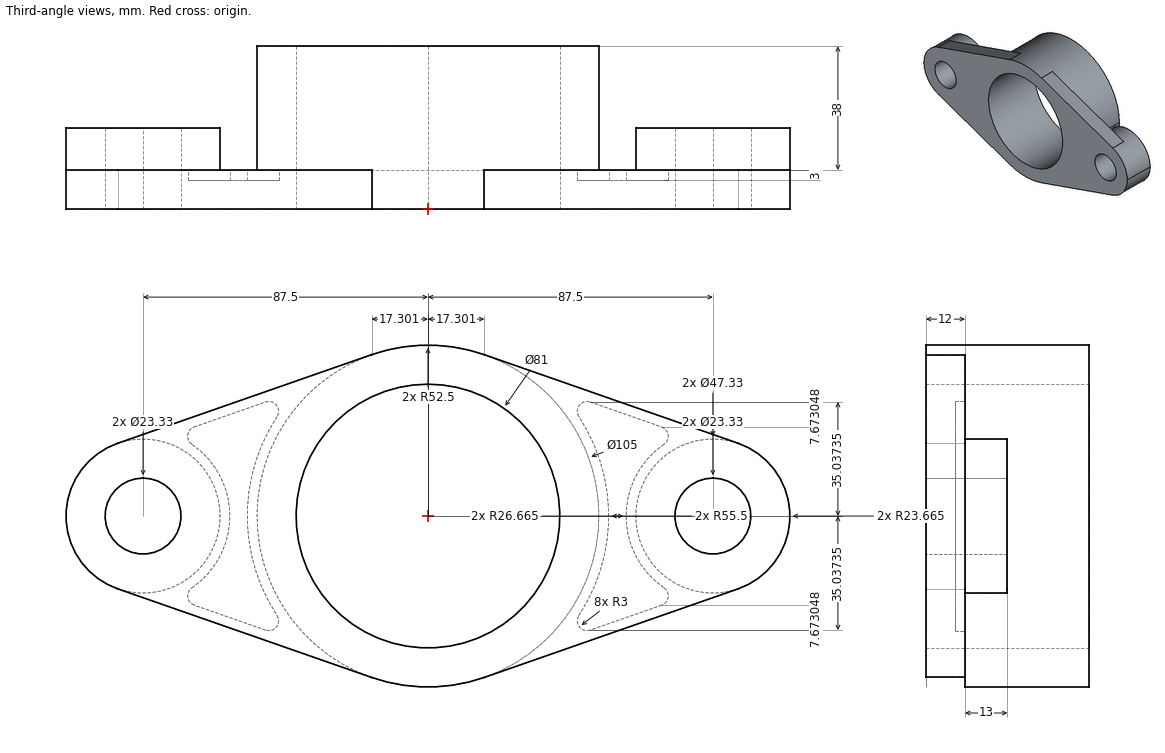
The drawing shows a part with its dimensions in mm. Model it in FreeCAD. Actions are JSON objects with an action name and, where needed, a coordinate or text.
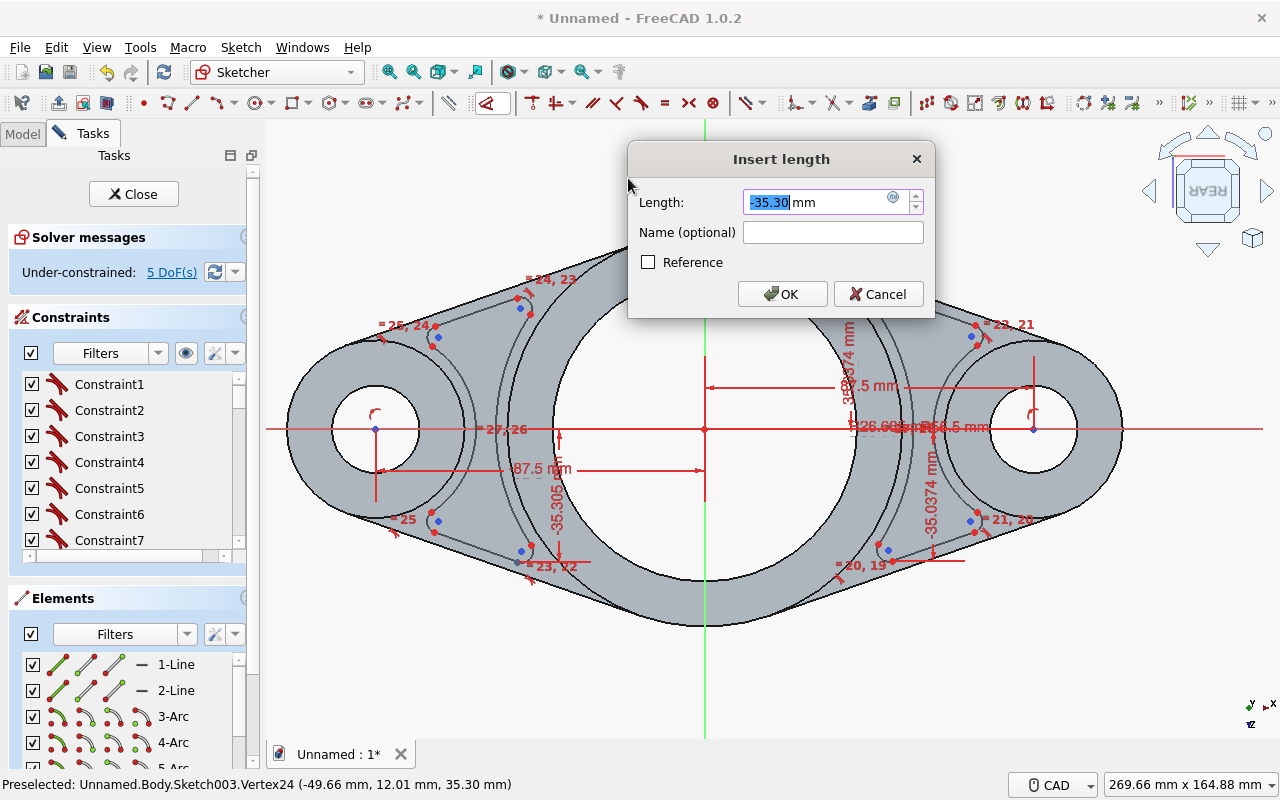
{"action": "type", "text": "-35.03735"}
{"action": "key", "text": "Return"}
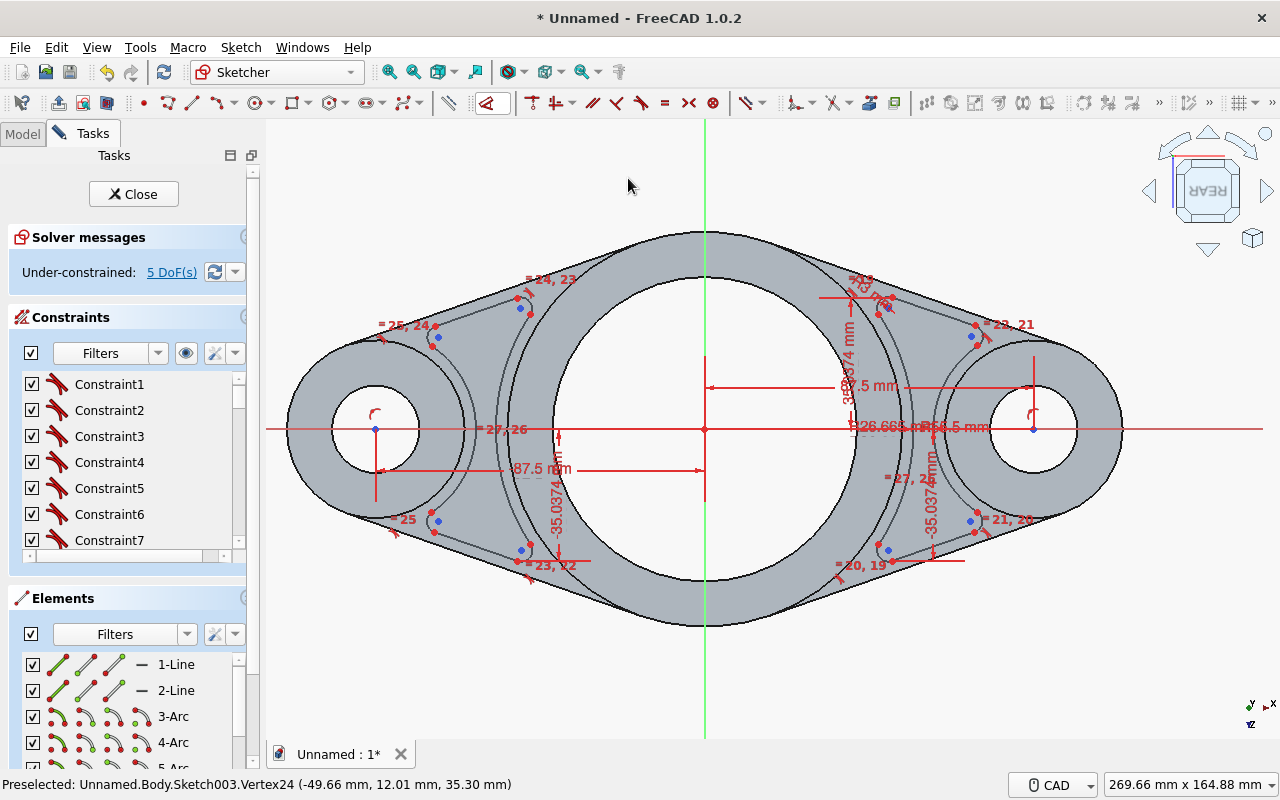
{"action": "left_click", "coordinate": [517, 298]}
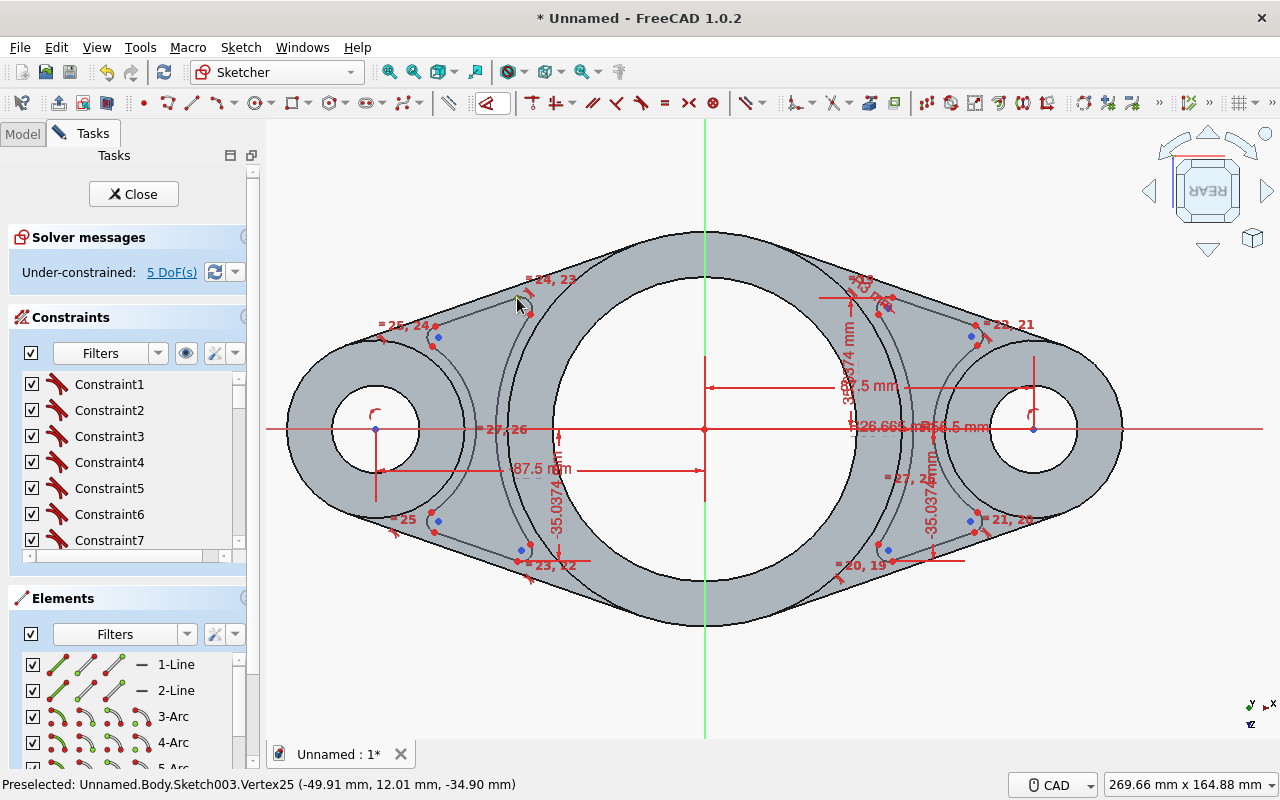
{"action": "left_click", "coordinate": [504, 104]}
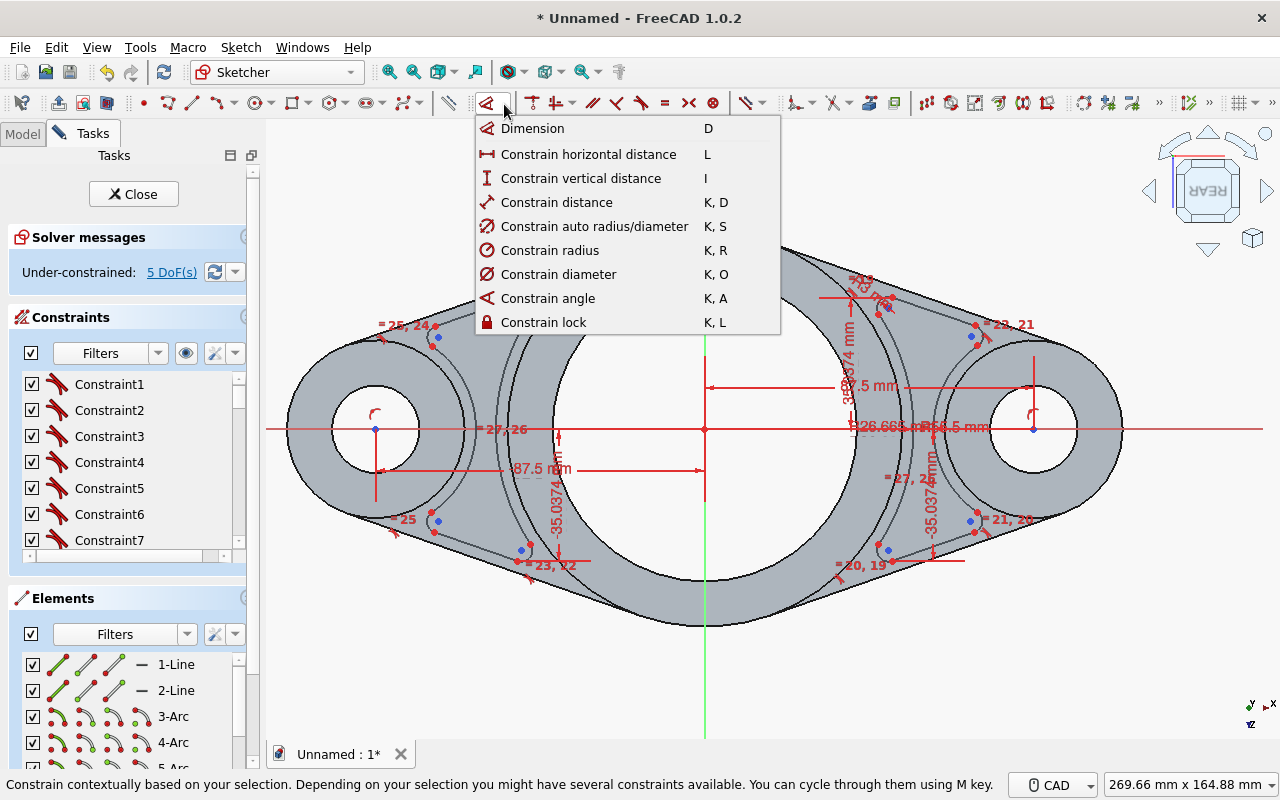
{"action": "left_click", "coordinate": [628, 178]}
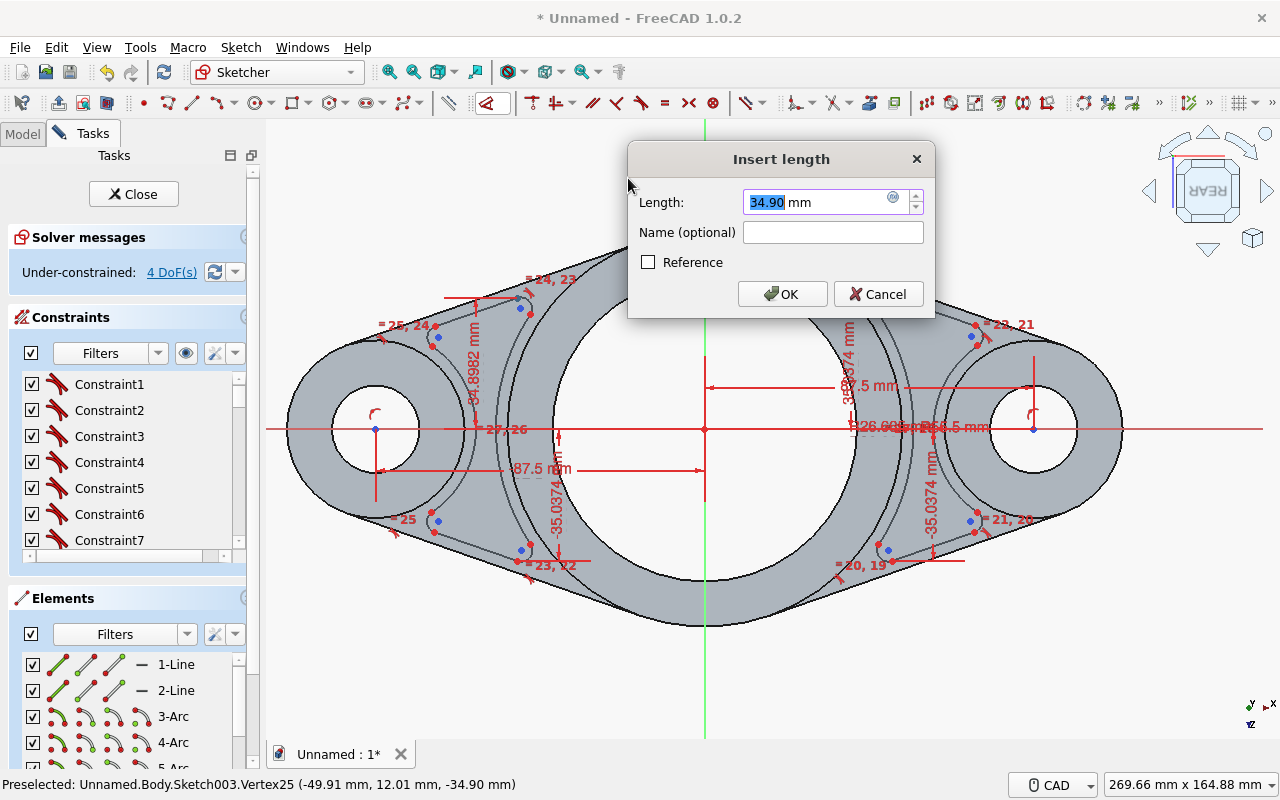
{"action": "type", "text": "35.03735"}
{"action": "key", "text": "Return"}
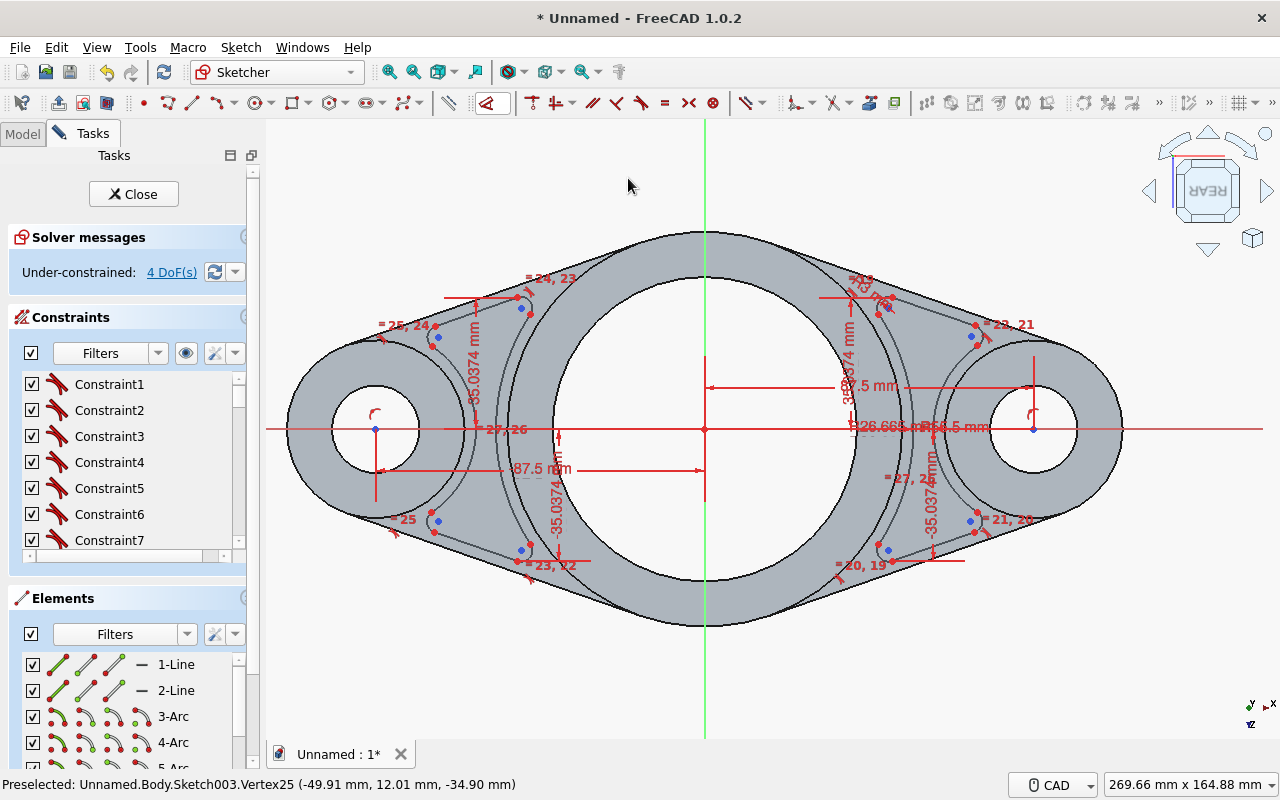
{"action": "scroll", "coordinate": [950, 317], "scroll_direction": "up", "scroll_amount": 2}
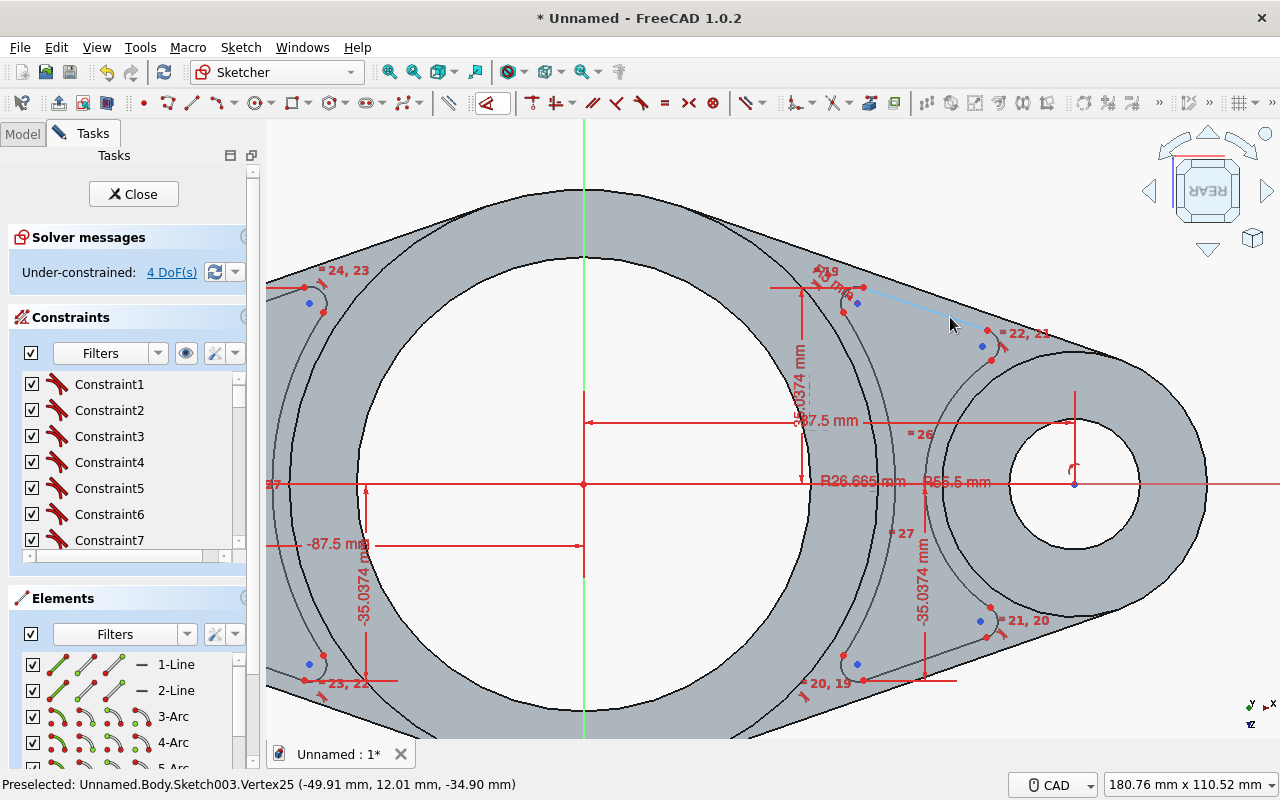
{"action": "left_click", "coordinate": [950, 317]}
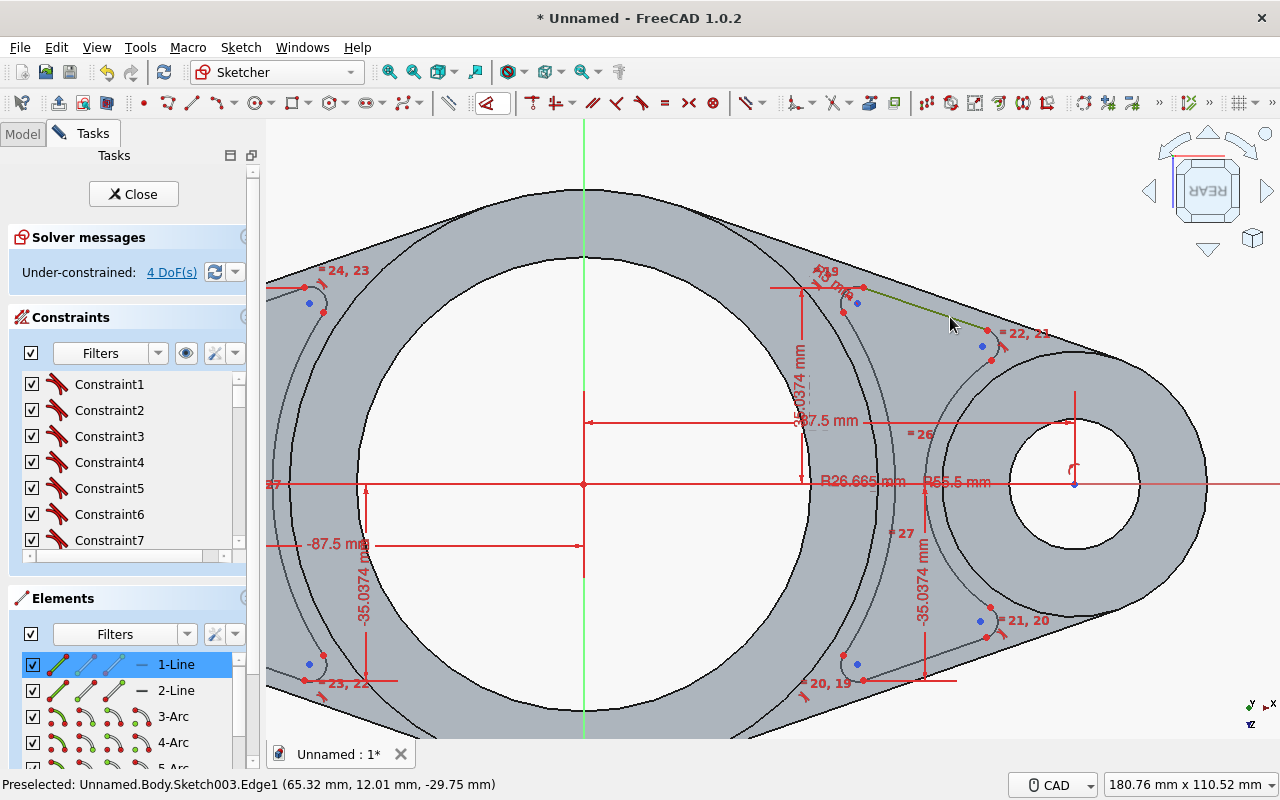
{"action": "left_click", "coordinate": [504, 104]}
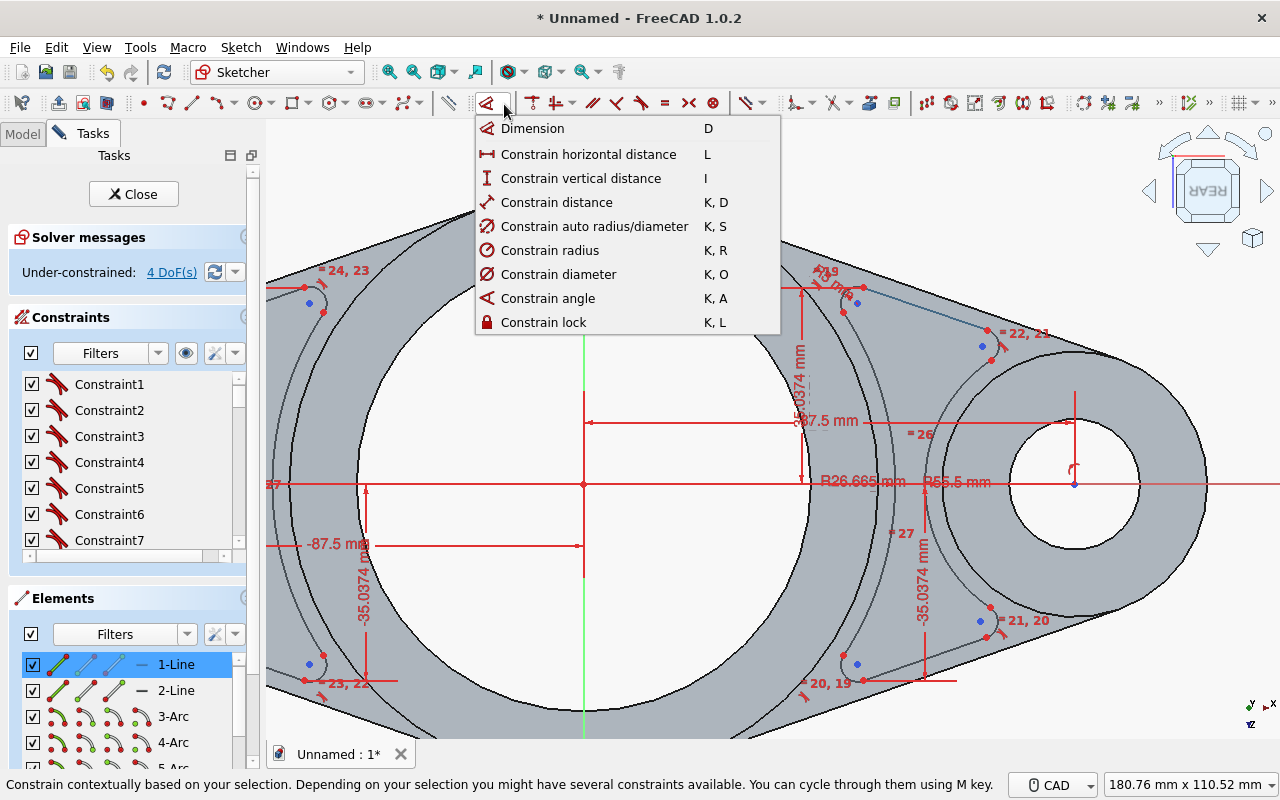
{"action": "left_click", "coordinate": [628, 178]}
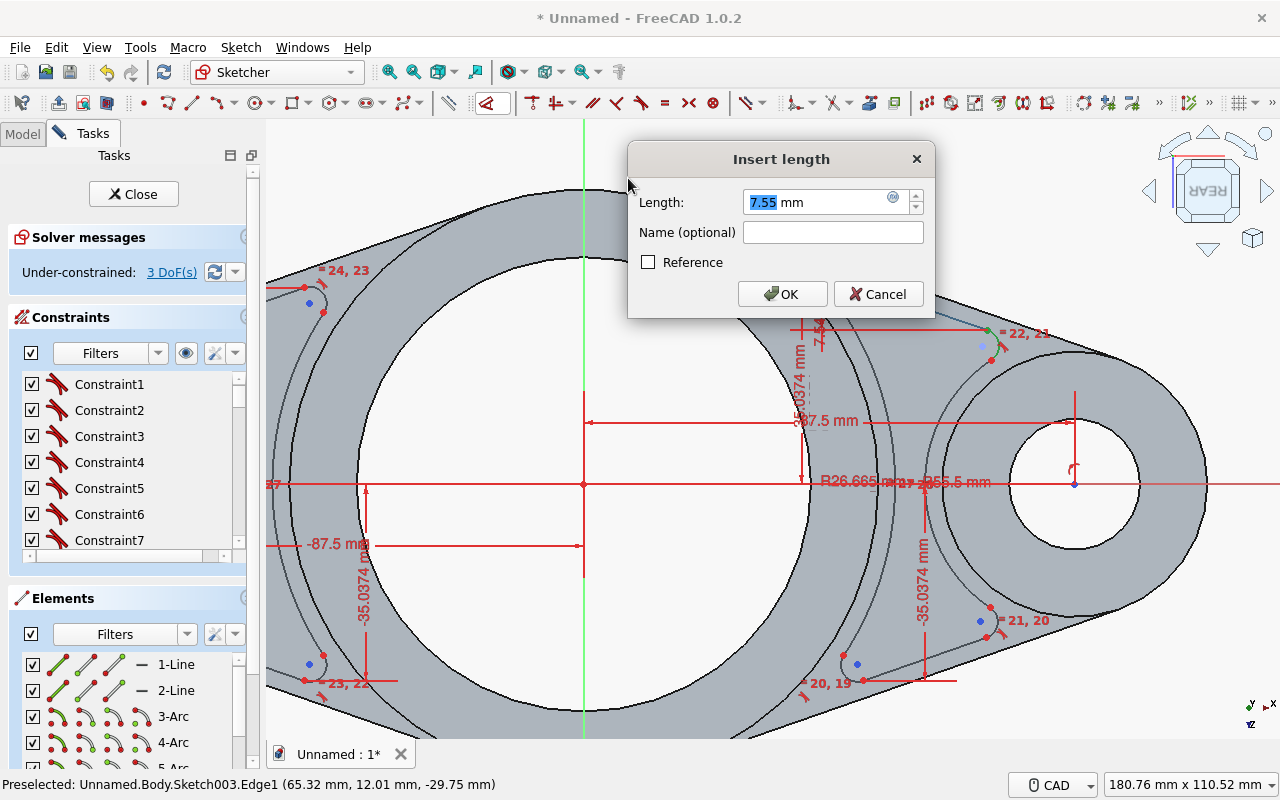
{"action": "type", "text": "7.673048"}
{"action": "key", "text": "Return"}